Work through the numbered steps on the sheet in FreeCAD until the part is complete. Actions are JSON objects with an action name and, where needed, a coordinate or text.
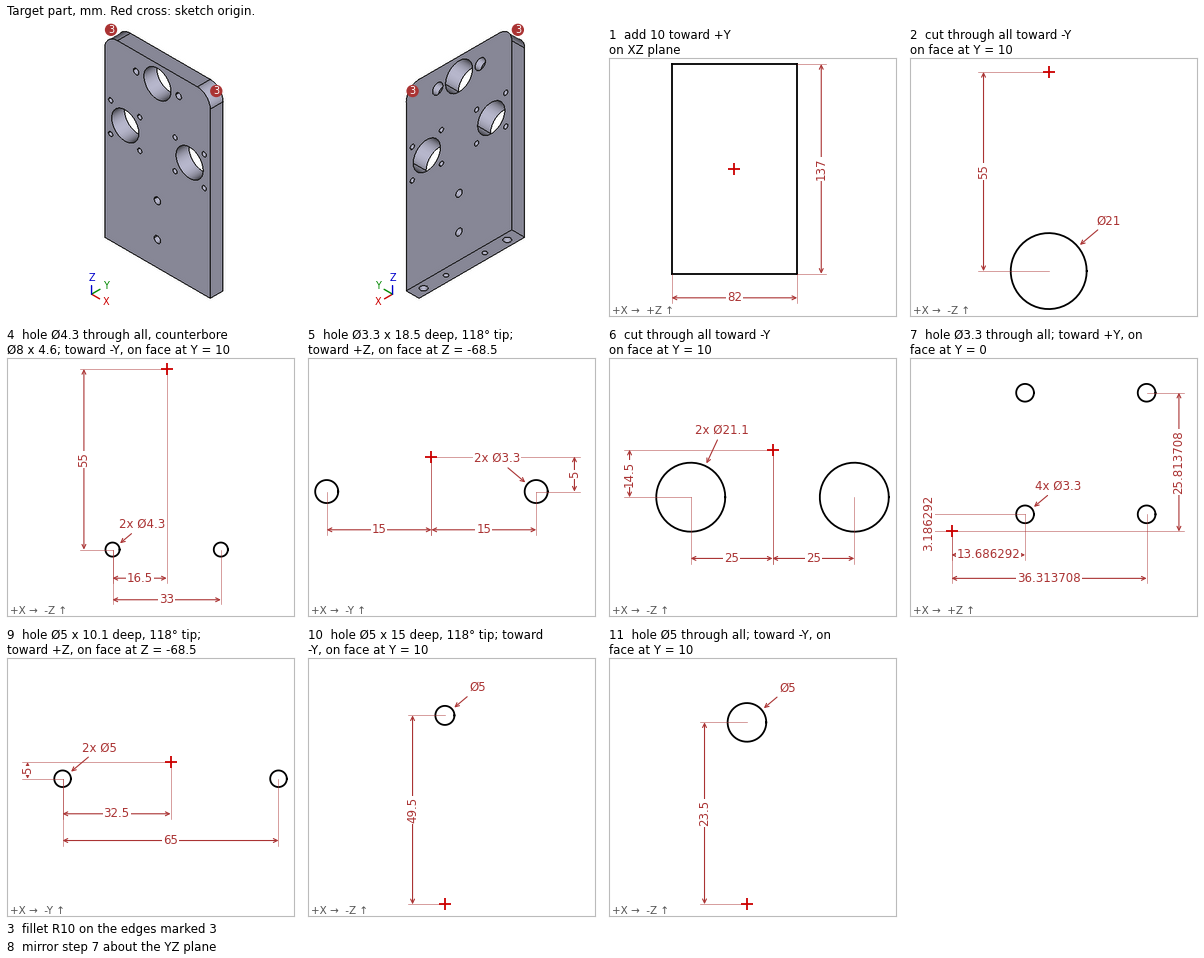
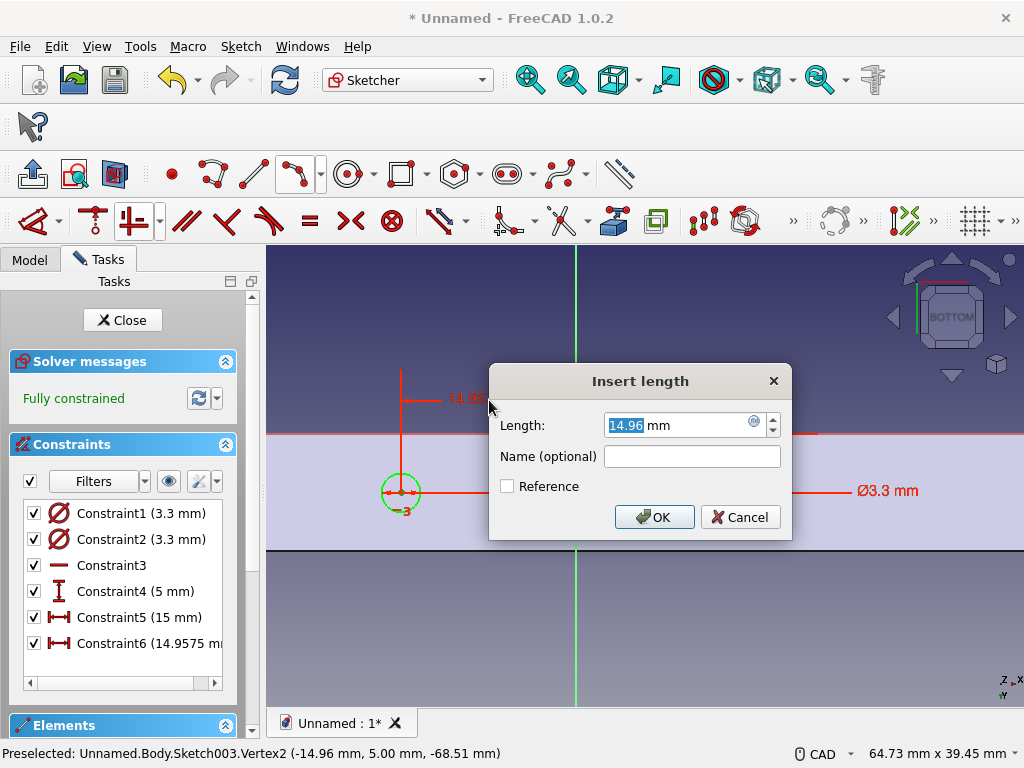
{"action": "type", "text": "15"}
{"action": "key", "text": "Return"}
{"action": "key", "text": "Escape"}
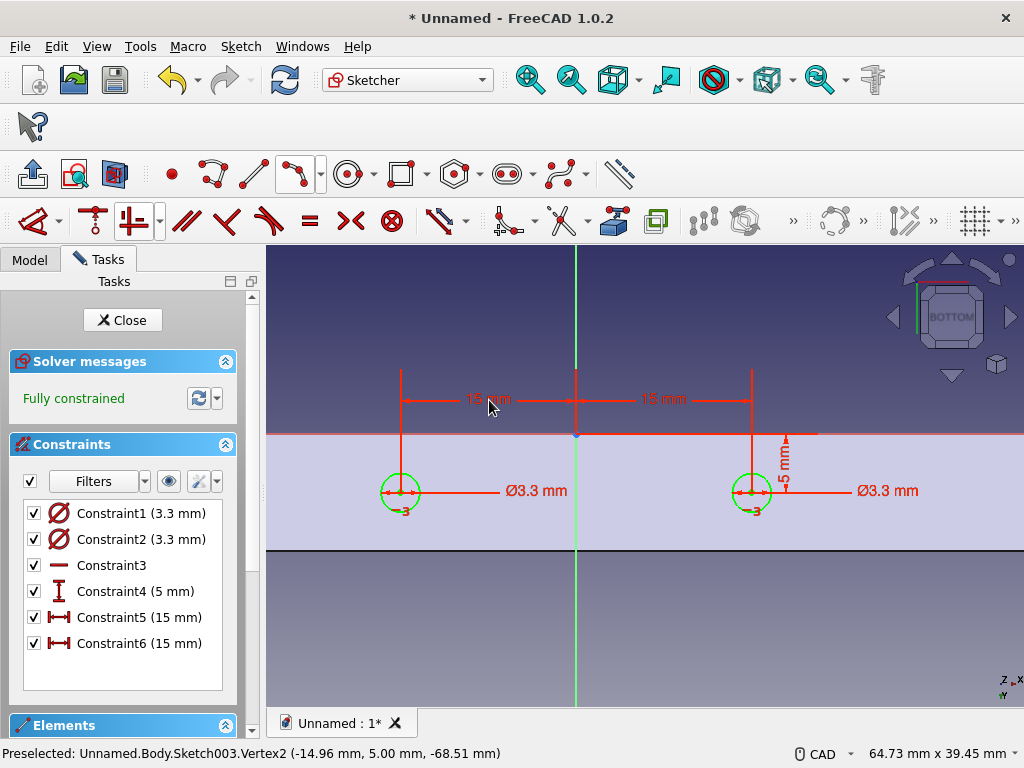
{"action": "left_click", "coordinate": [123, 320]}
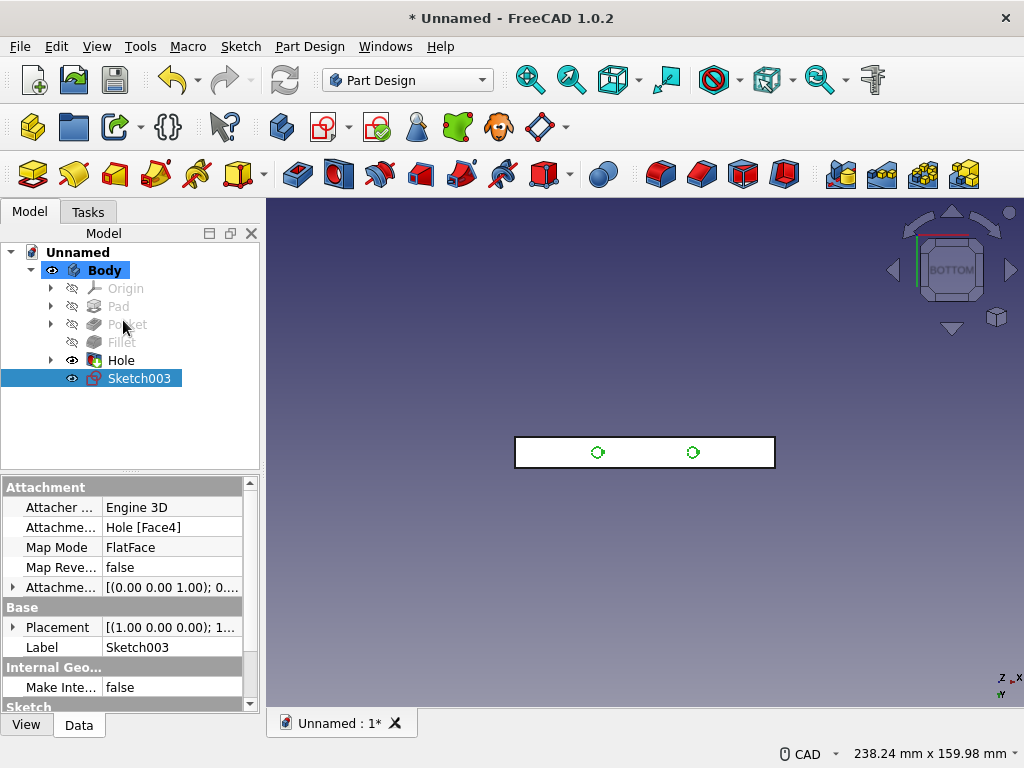
{"action": "left_click", "coordinate": [339, 174]}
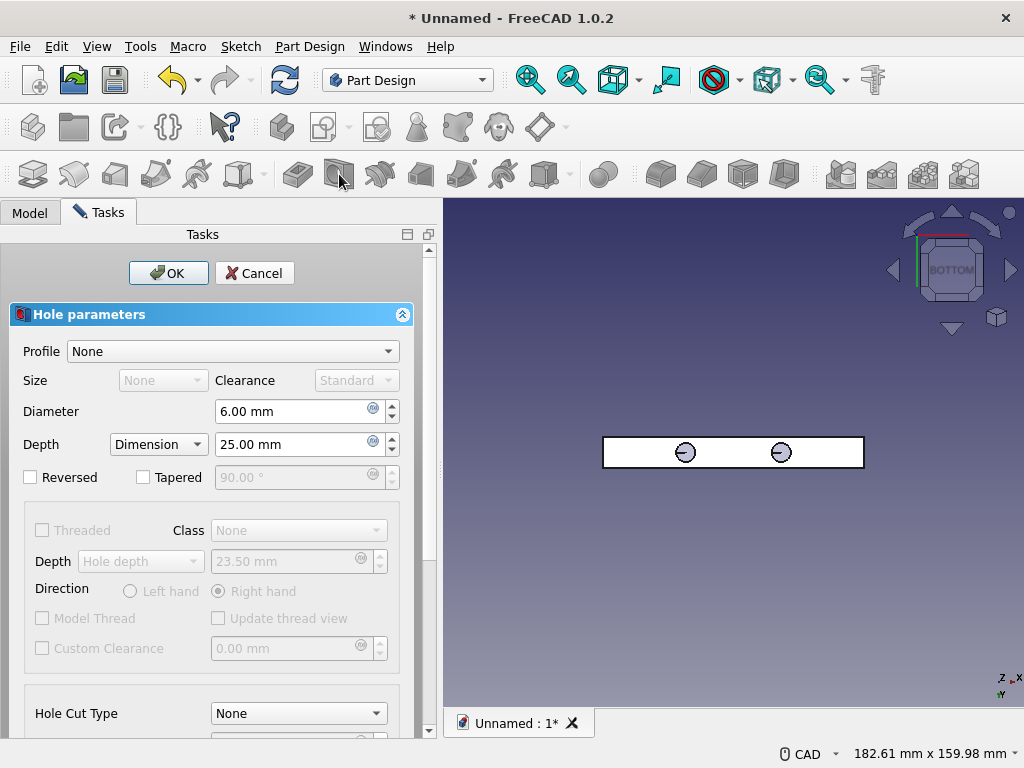
{"action": "triple_click", "coordinate": [300, 412]}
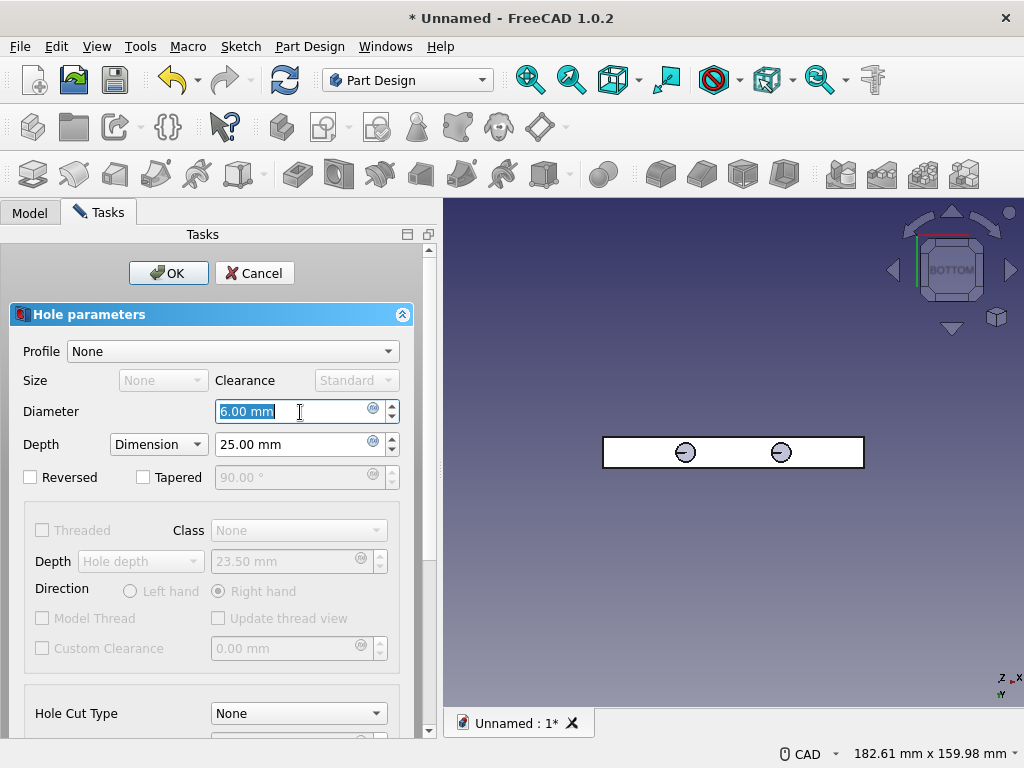
{"action": "type", "text": "3.3"}
{"action": "key", "text": "Tab"}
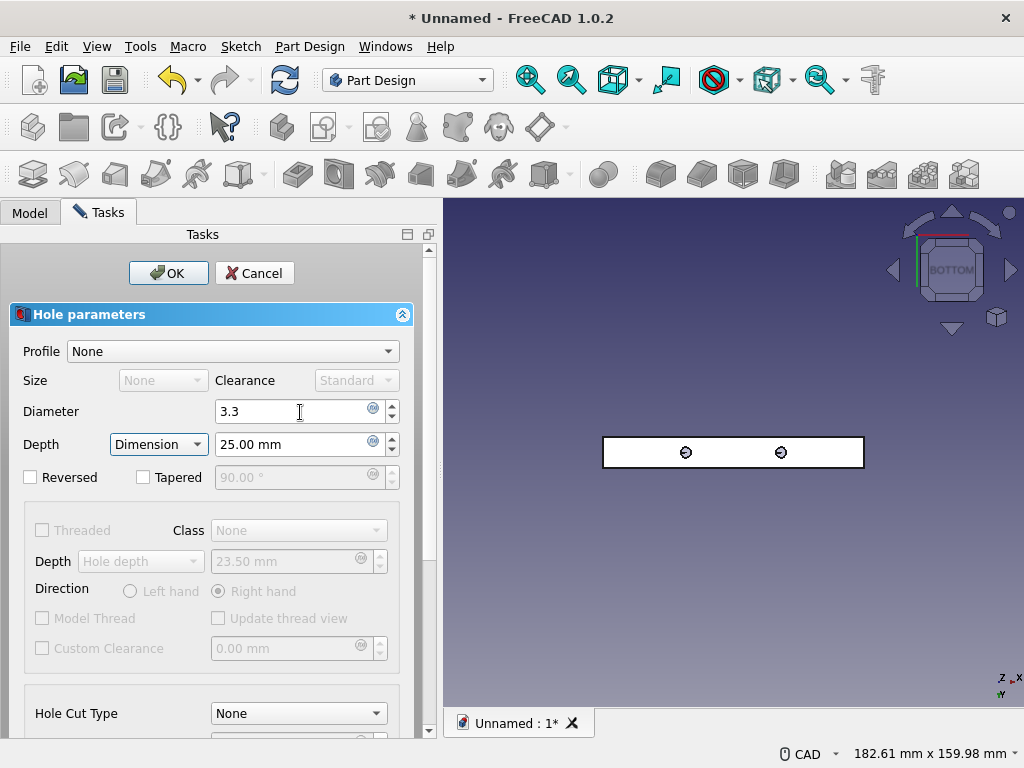
{"action": "triple_click", "coordinate": [300, 444]}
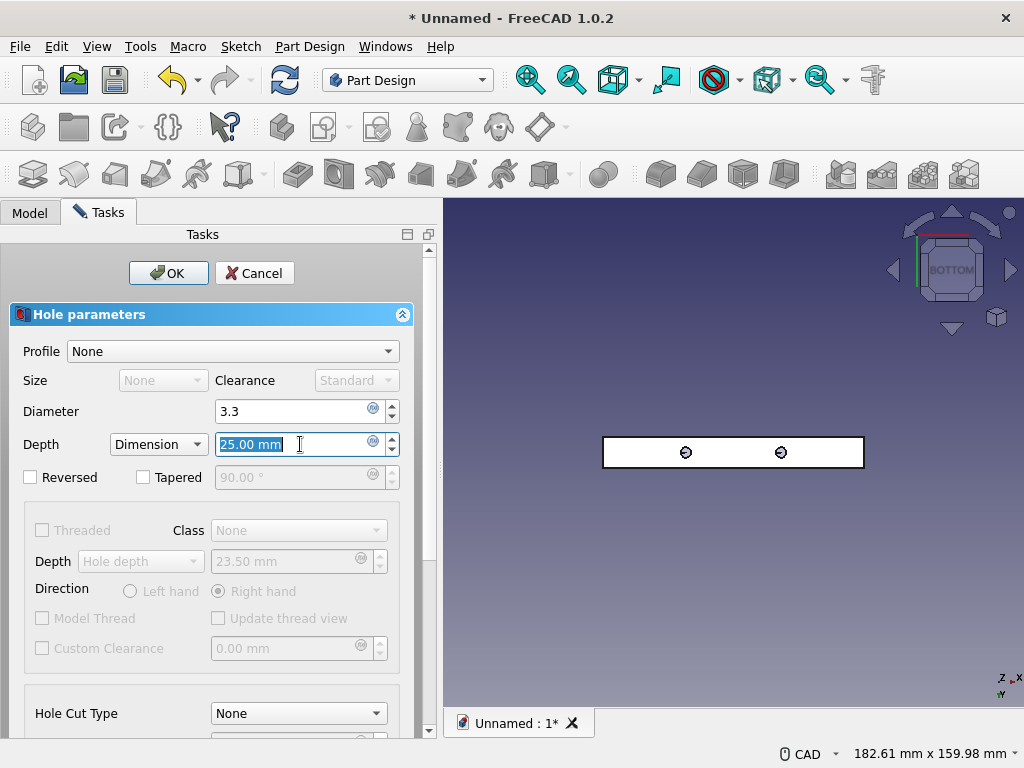
{"action": "type", "text": "18.5"}
{"action": "key", "text": "Tab"}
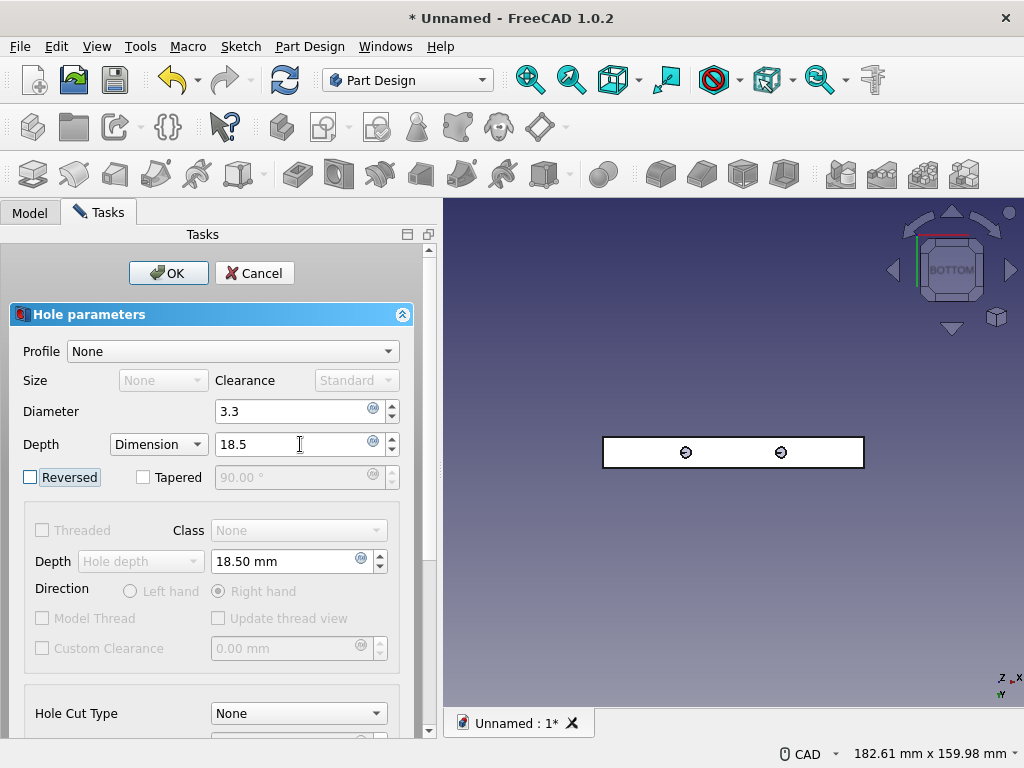
{"action": "left_click", "coordinate": [169, 273]}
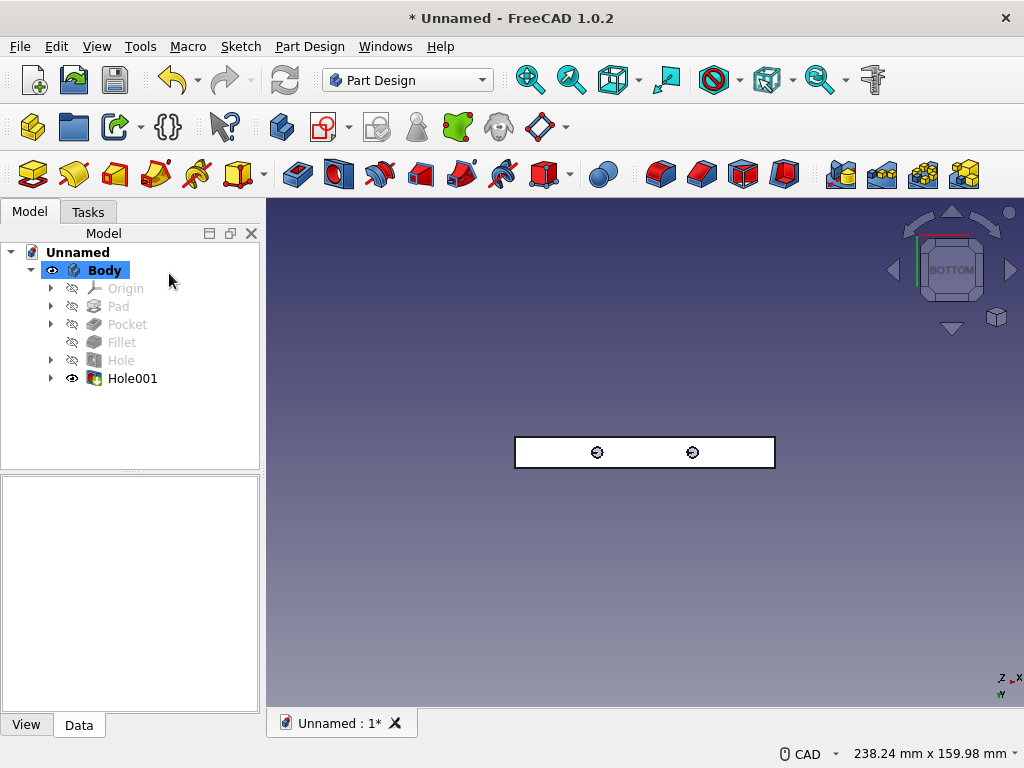
{"action": "left_click", "coordinate": [531, 80]}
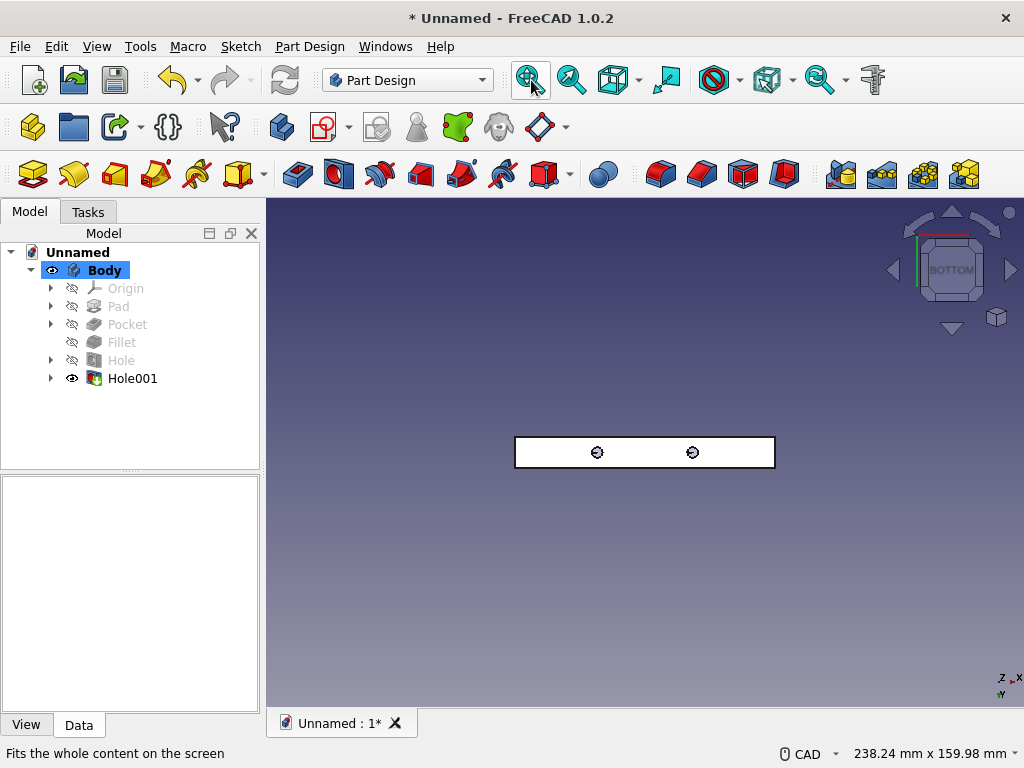
{"action": "key", "text": "4"}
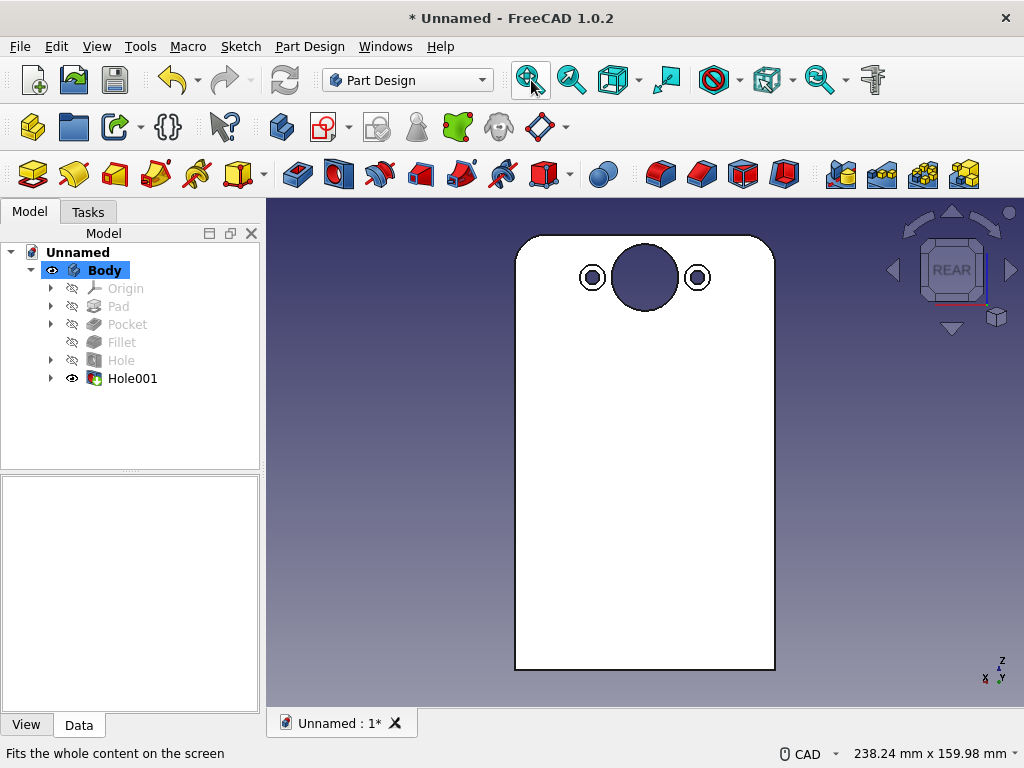
{"action": "left_click", "coordinate": [645, 451]}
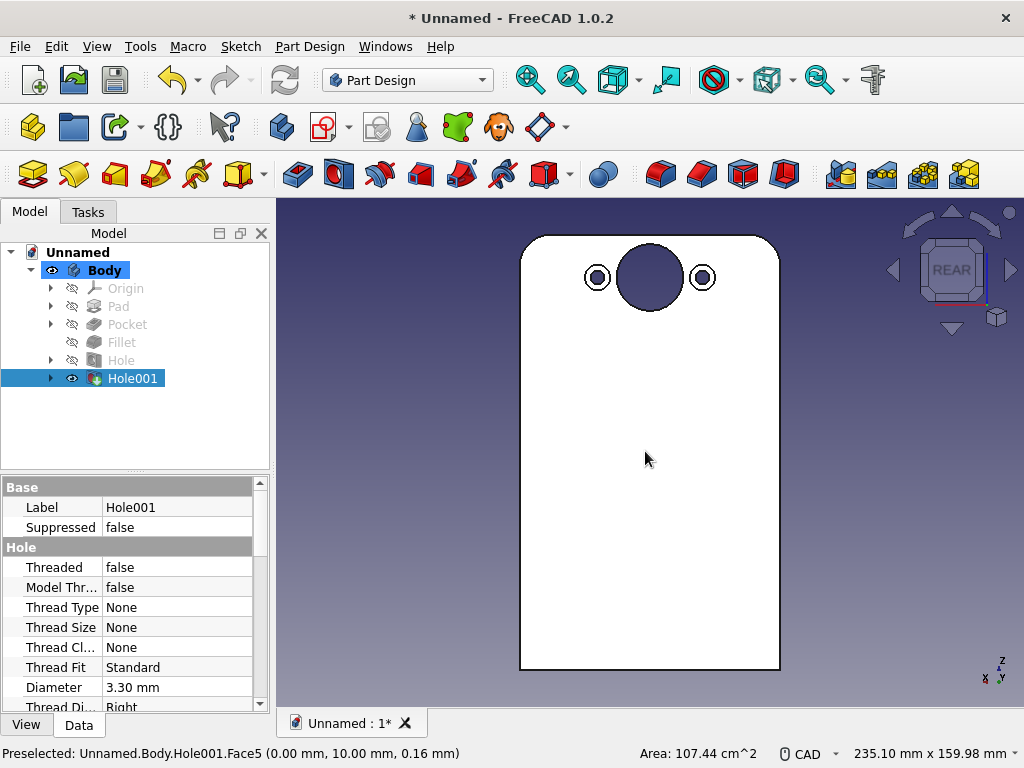
{"action": "left_click", "coordinate": [322, 128]}